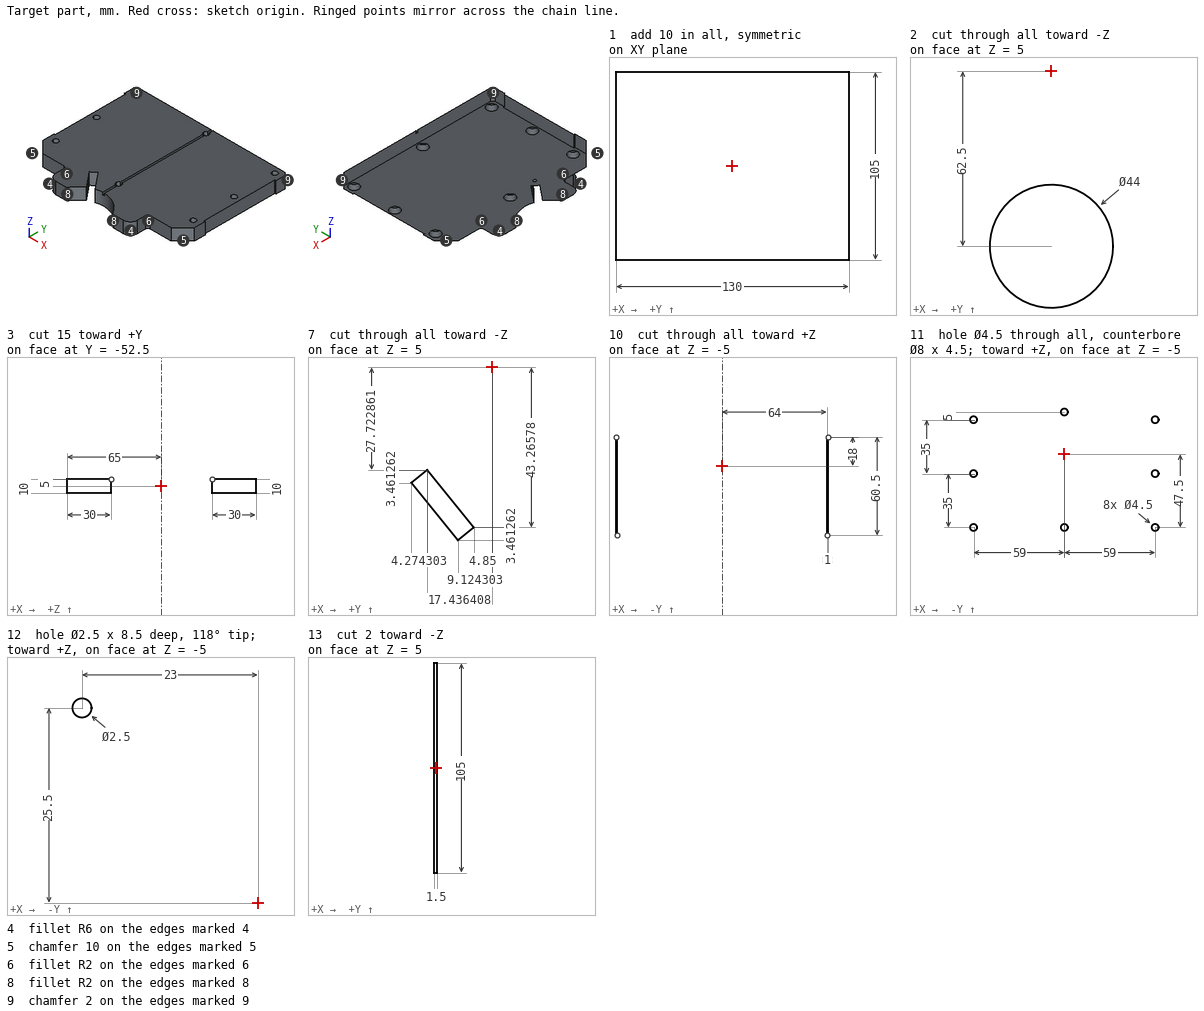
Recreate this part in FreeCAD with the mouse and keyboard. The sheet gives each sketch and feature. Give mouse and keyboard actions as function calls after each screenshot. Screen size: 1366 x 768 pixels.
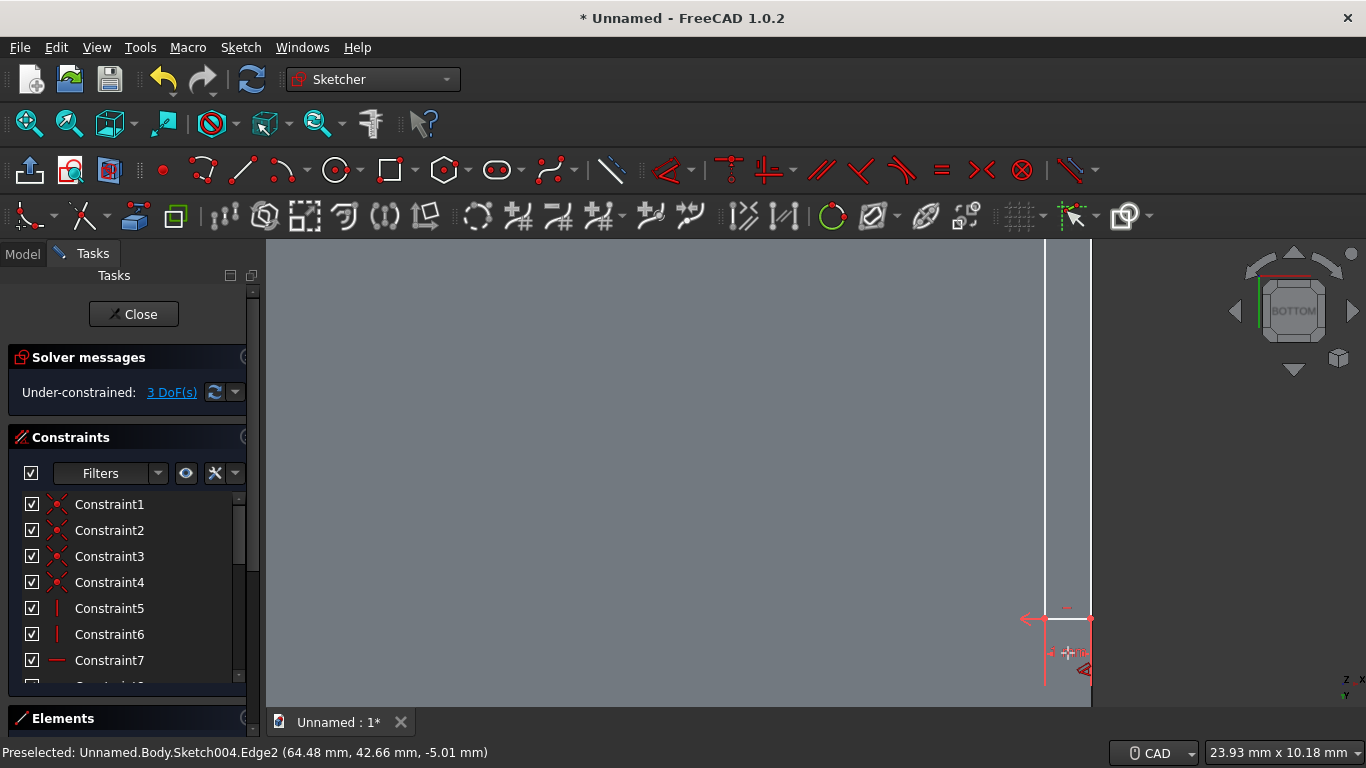
scroll(1077, 629, down, 11)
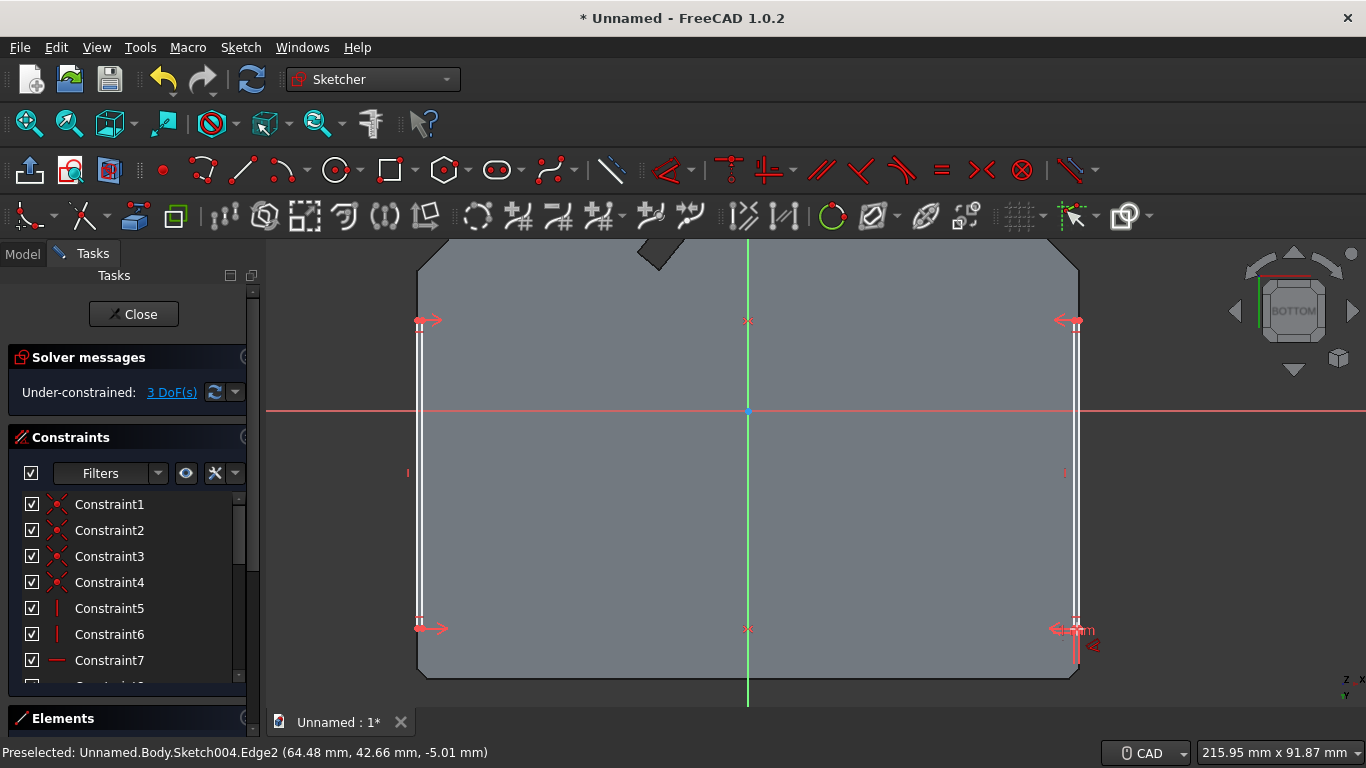
scroll(1074, 320, up, 5)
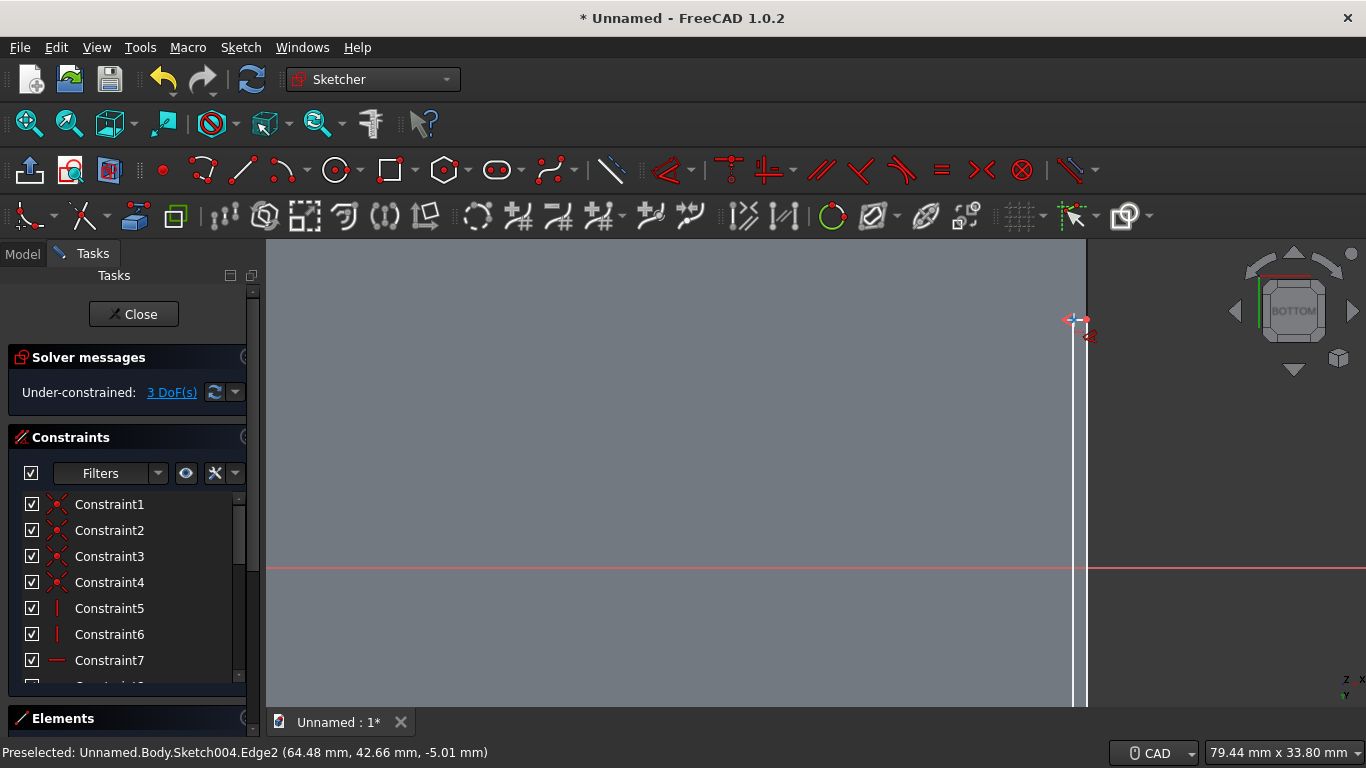
click(1073, 320)
click(684, 286)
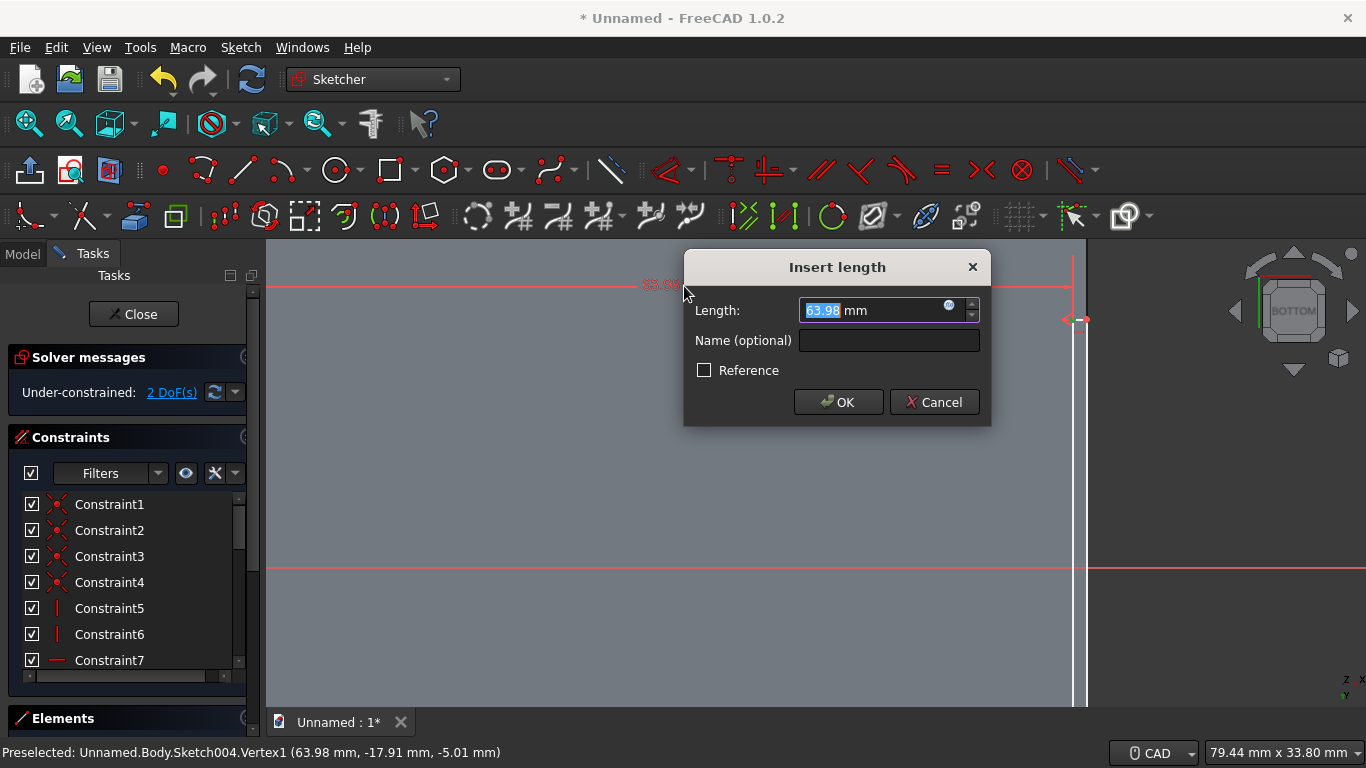
text(64)
key(Return)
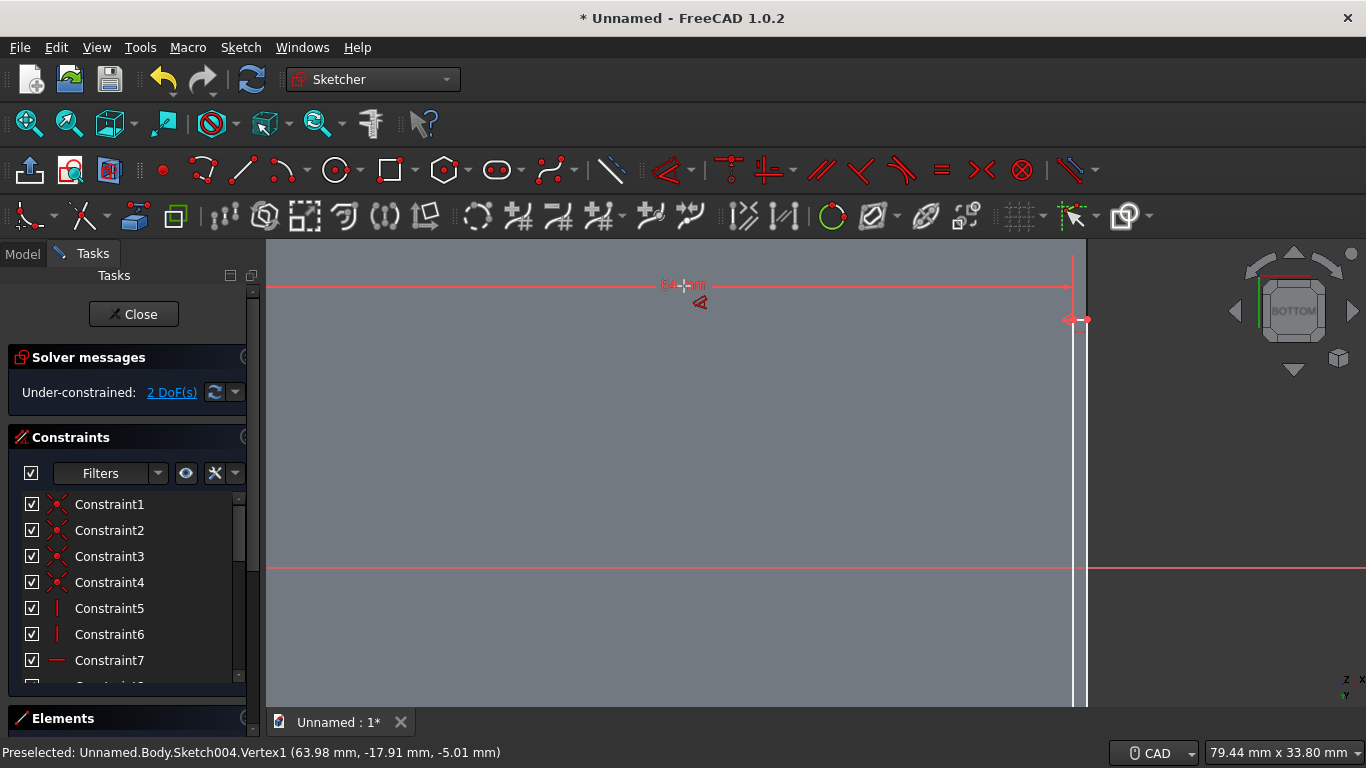
click(1073, 320)
click(1107, 444)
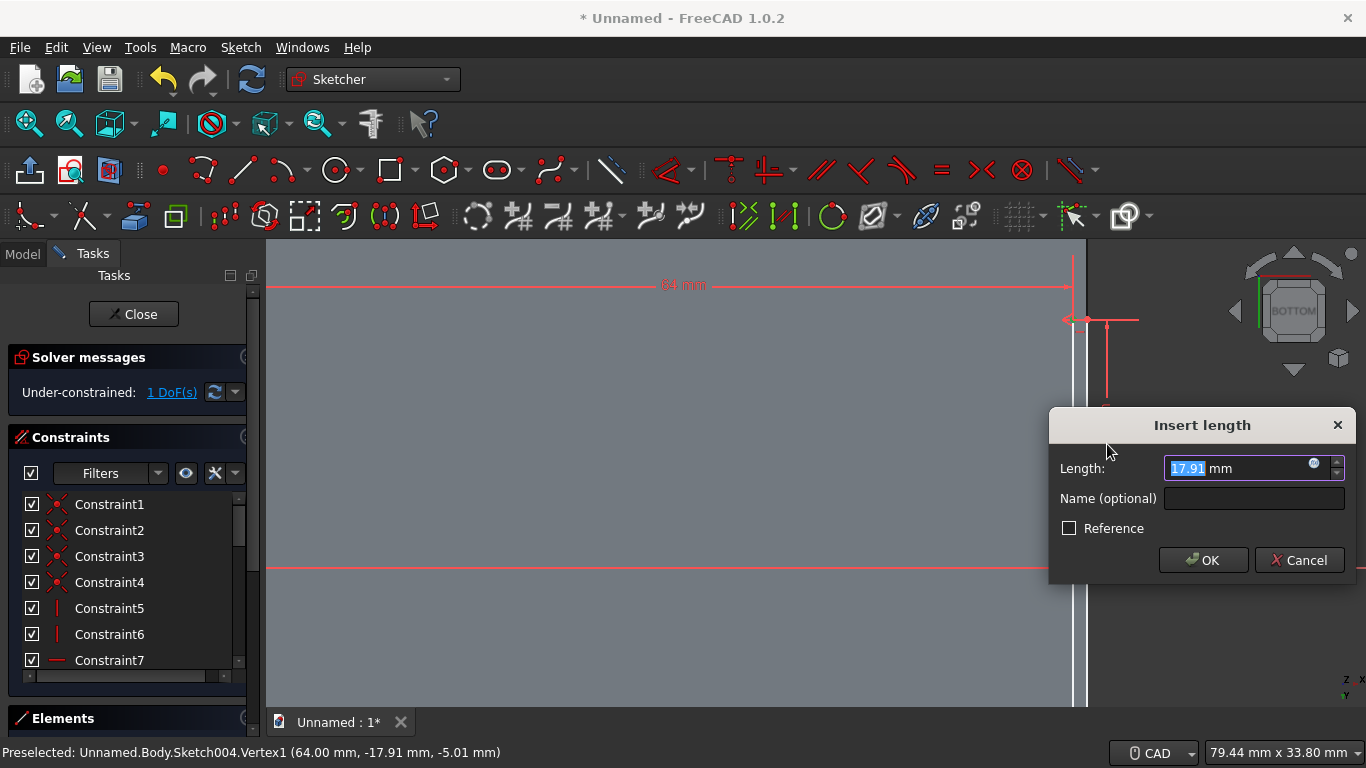
text(18)
key(Return)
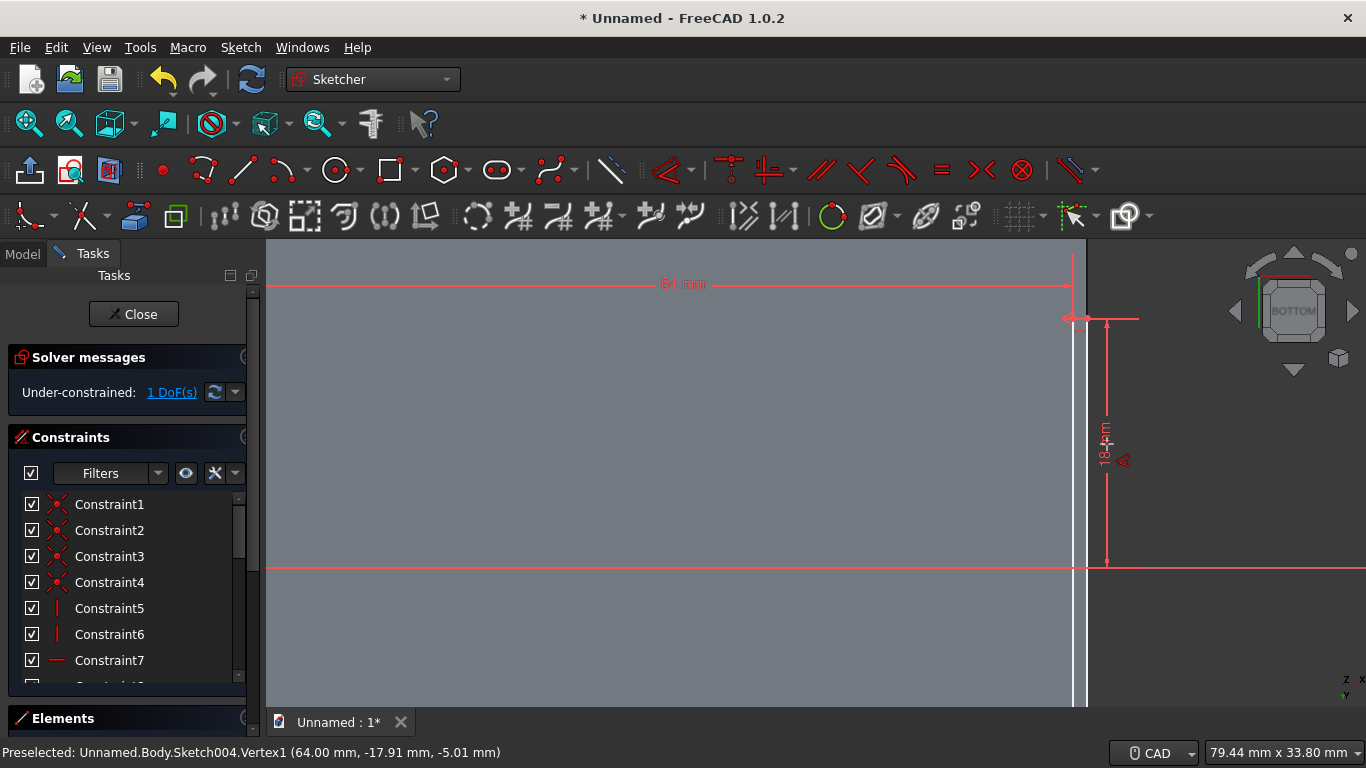
click(1073, 571)
click(1107, 499)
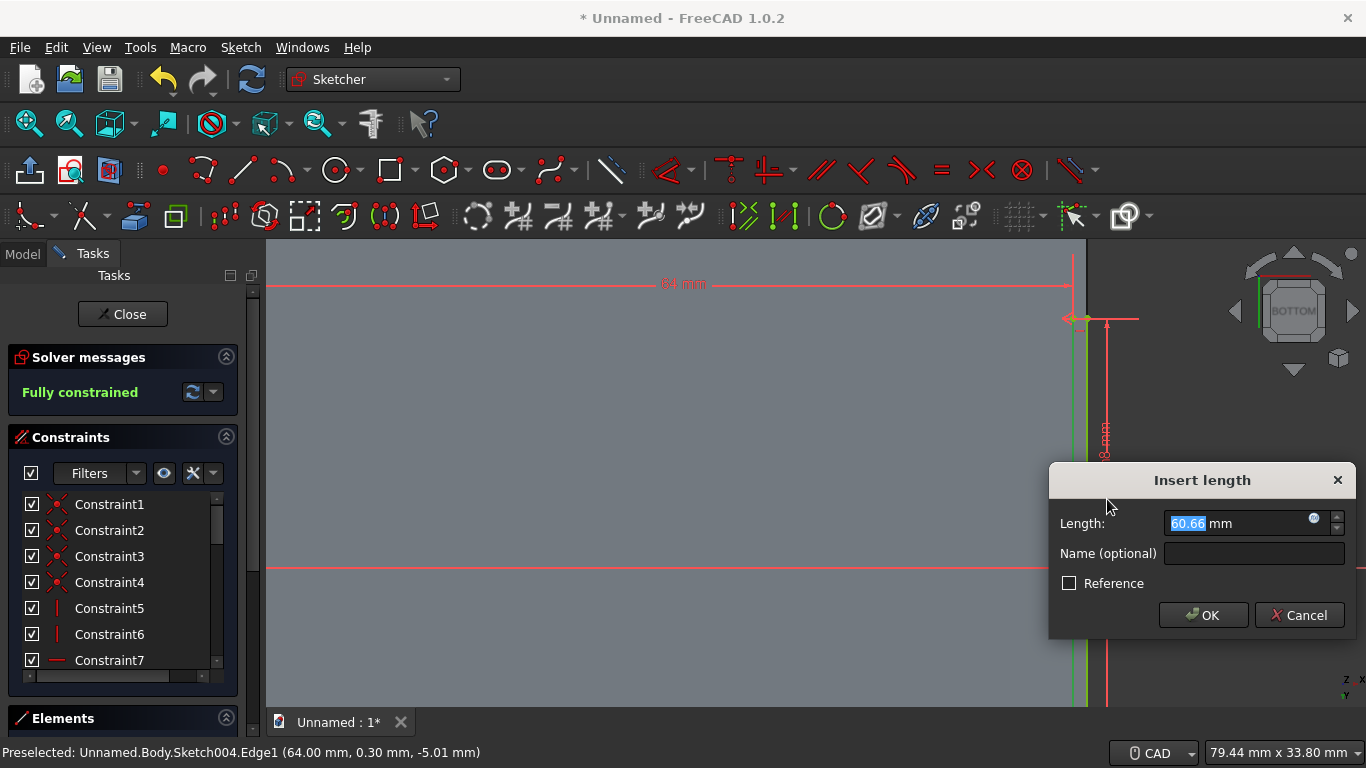
text(60.5)
key(Return)
key(Escape)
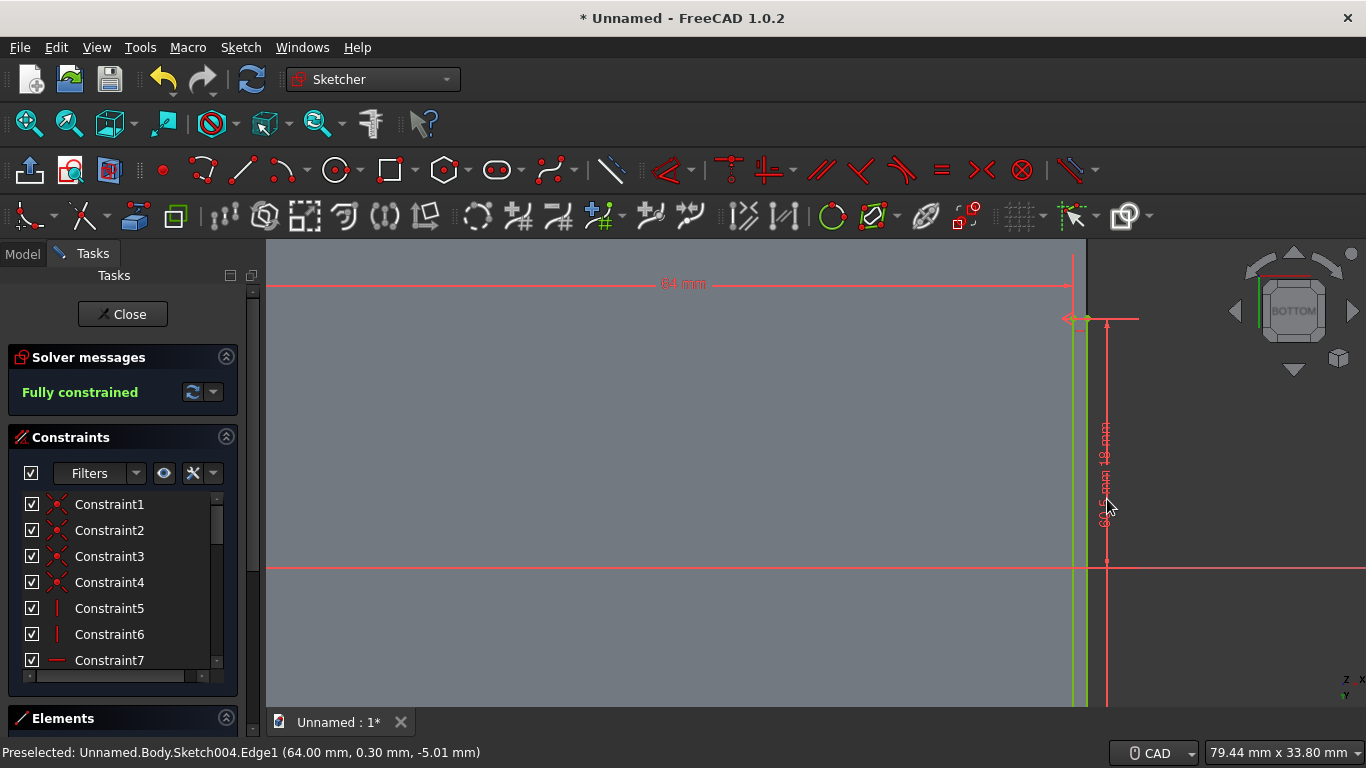
click(123, 314)